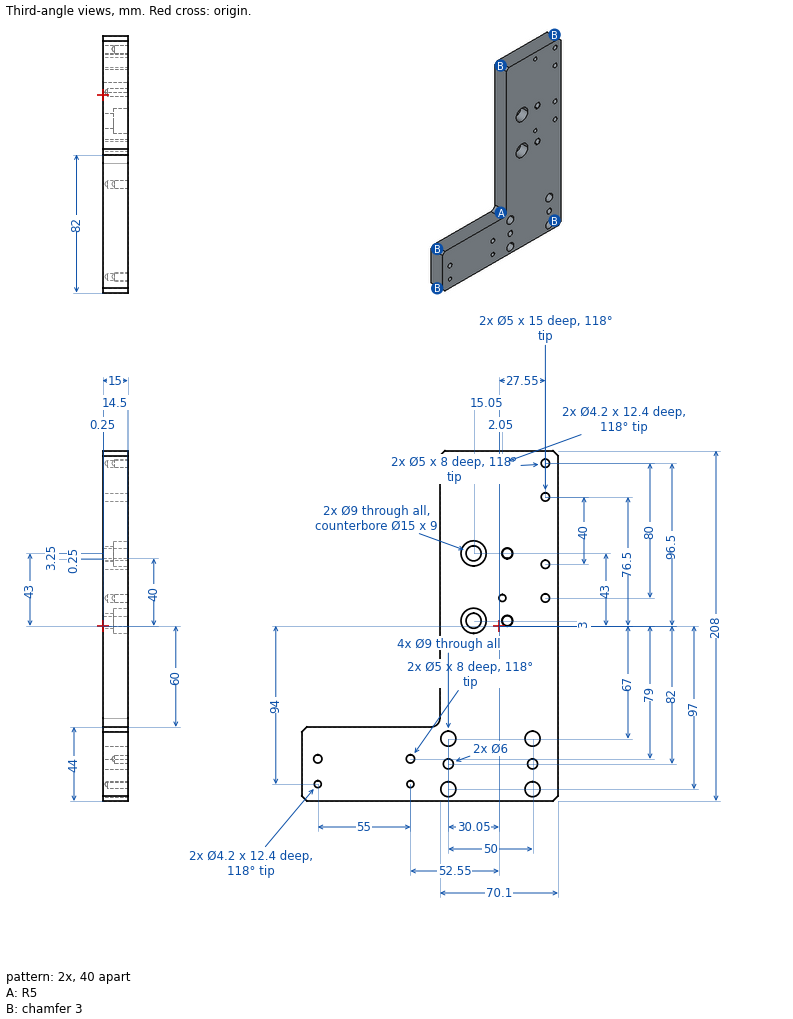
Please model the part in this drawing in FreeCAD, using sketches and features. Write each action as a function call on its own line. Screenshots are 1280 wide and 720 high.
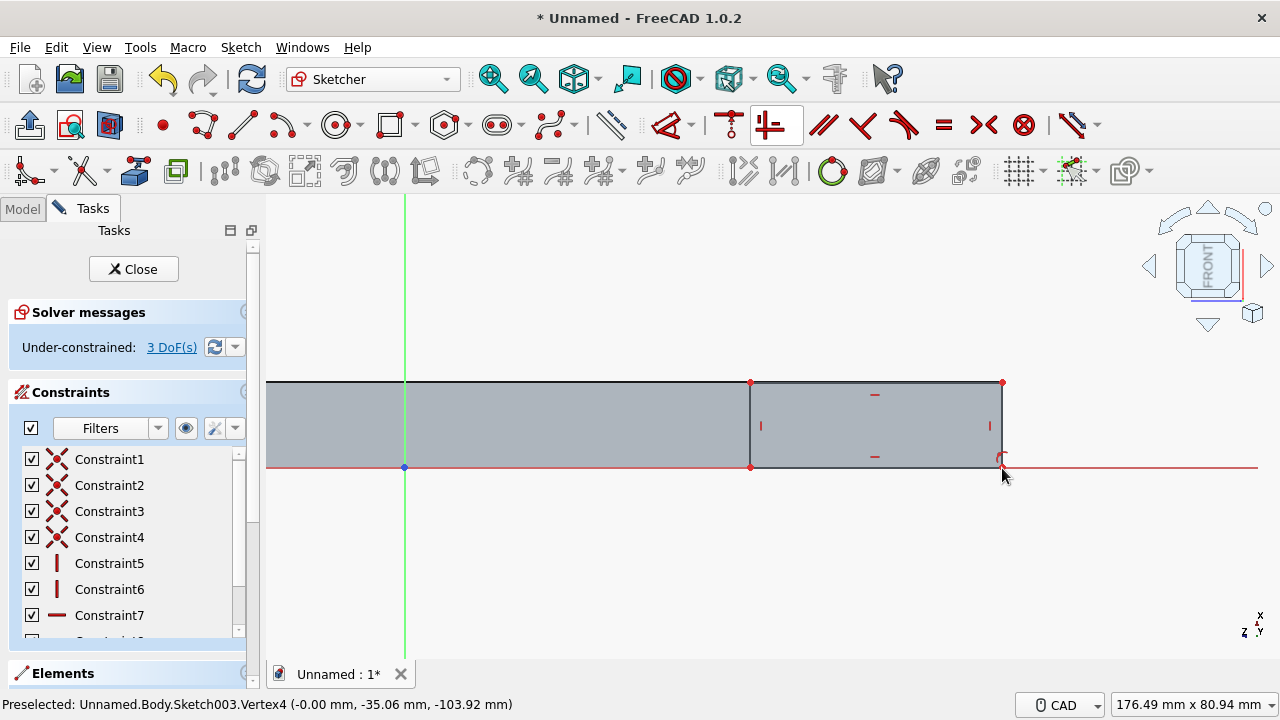
key(d)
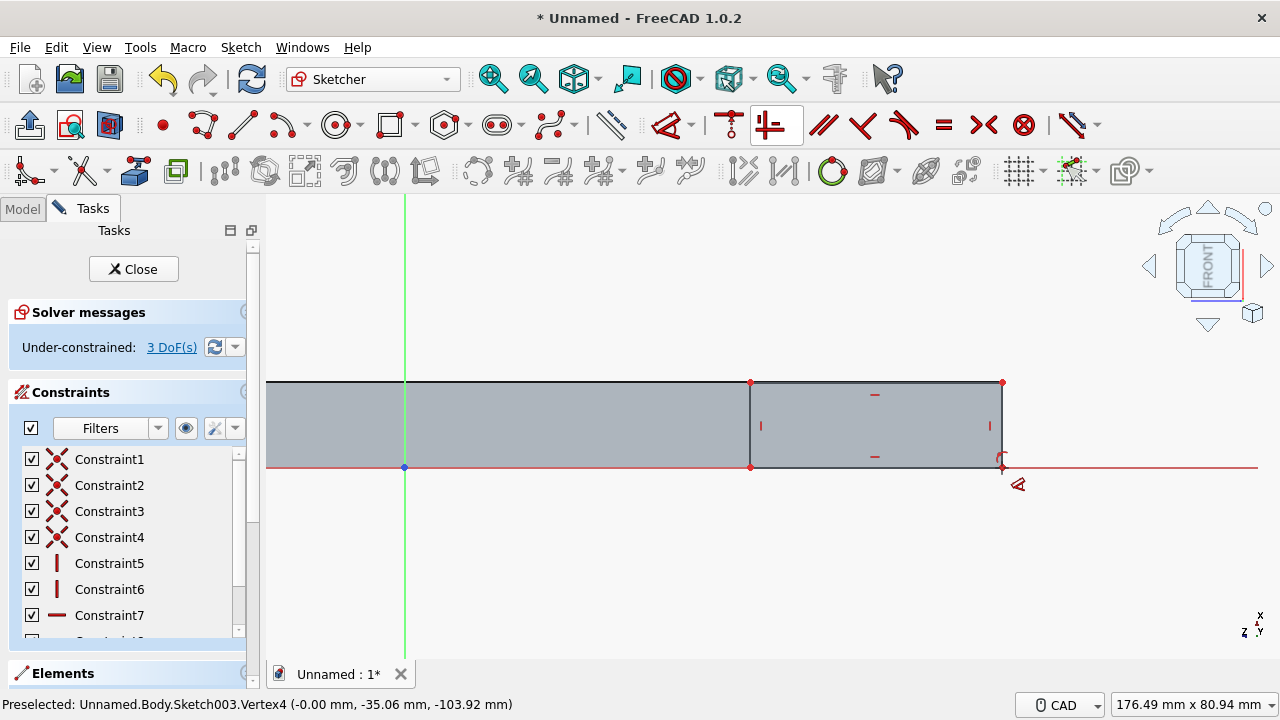
click(750, 408)
click(784, 425)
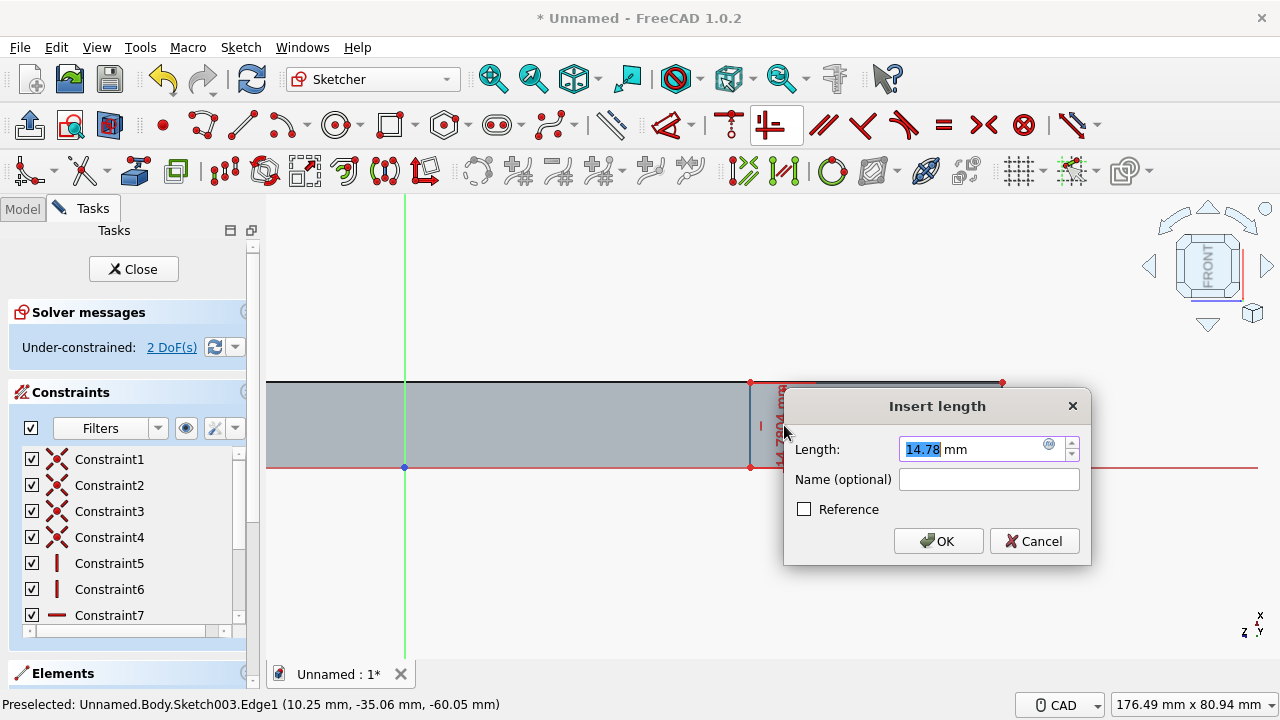
text(15)
key(Return)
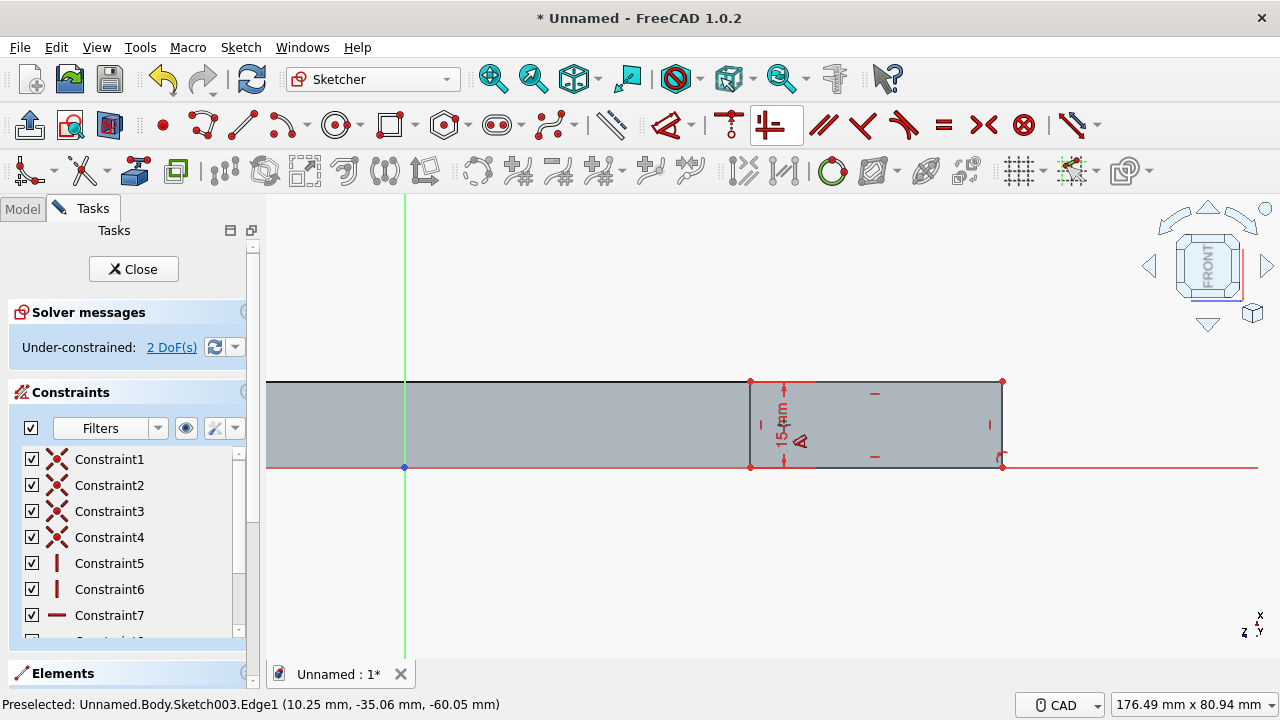
click(826, 468)
click(876, 502)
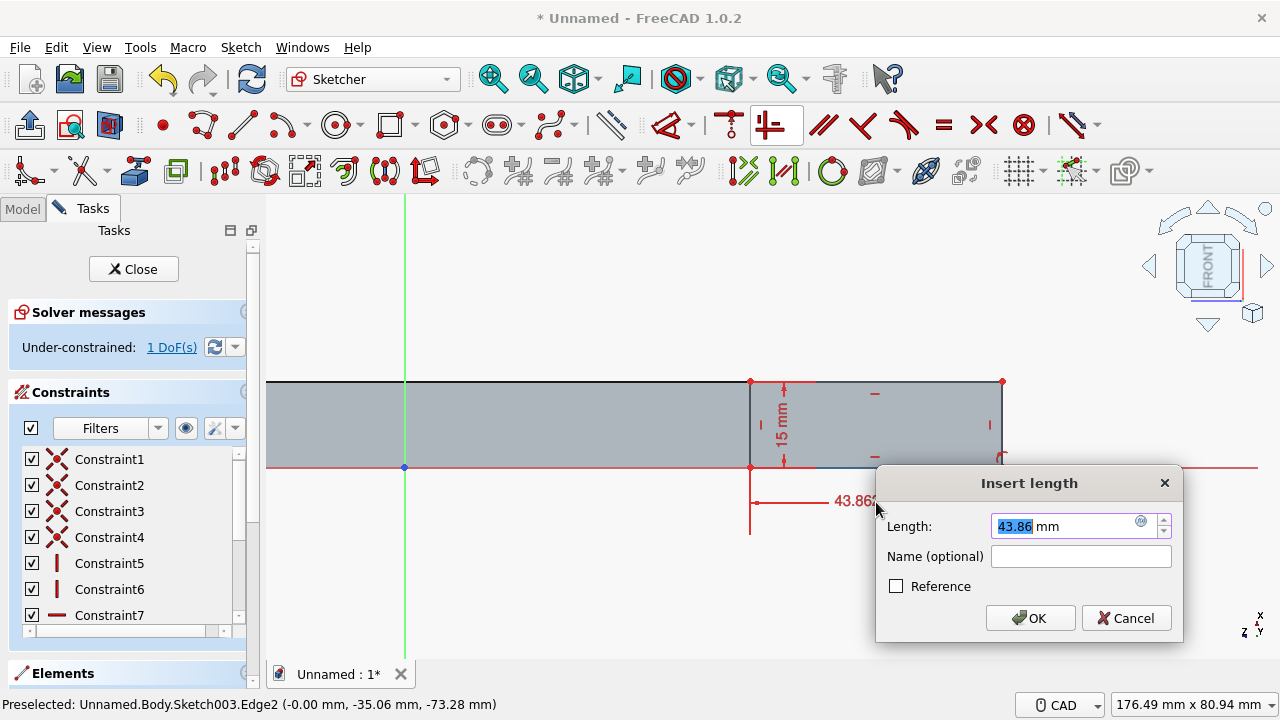
text(44)
key(Return)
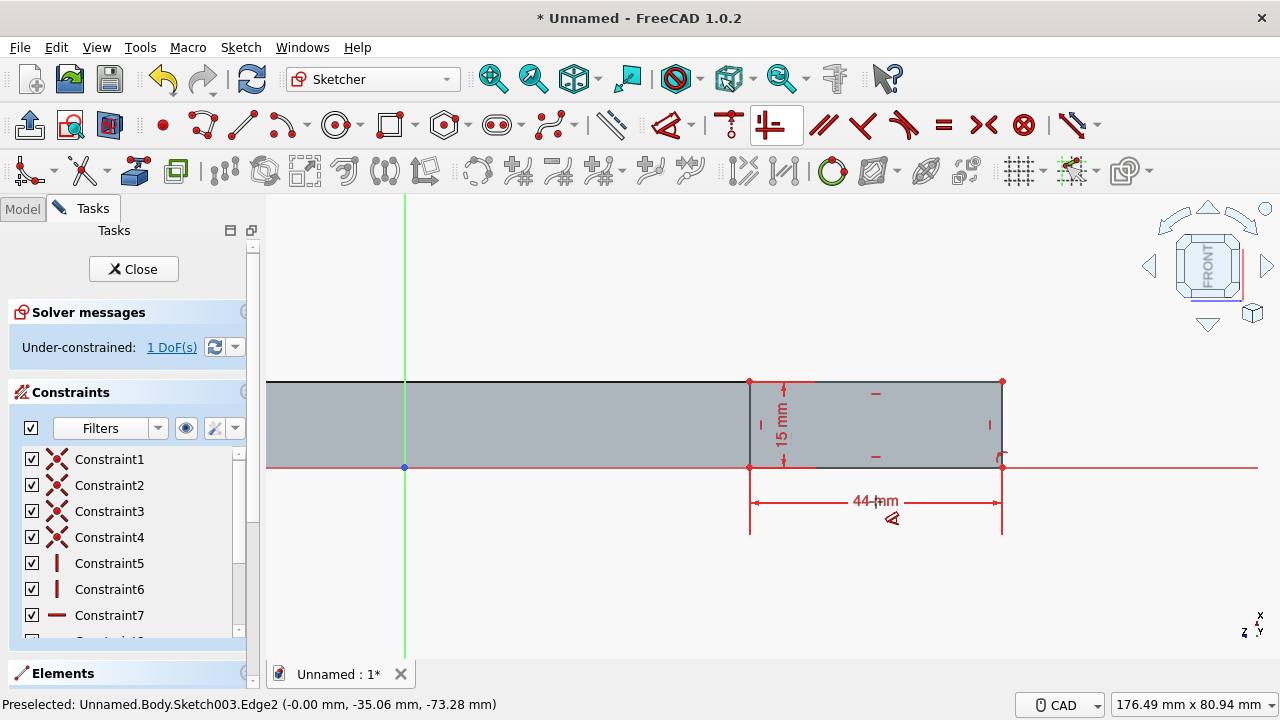
click(750, 382)
click(577, 502)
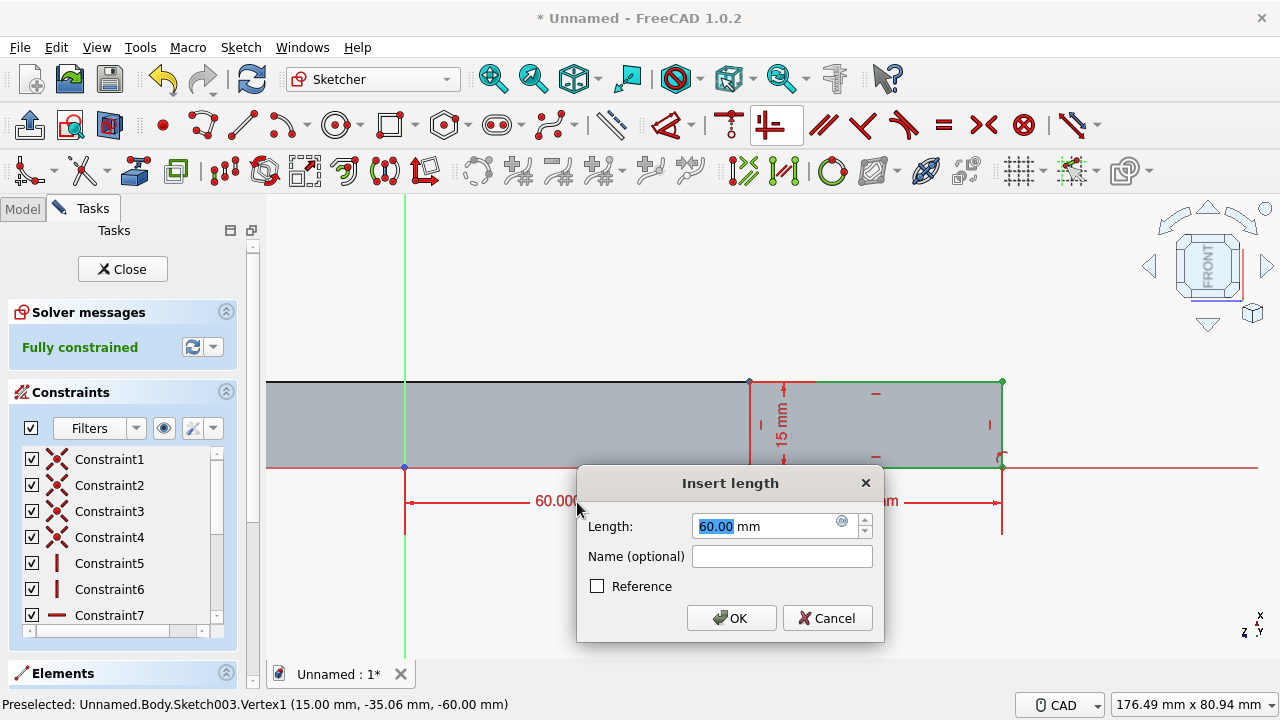
text(60)
key(Return)
key(Escape)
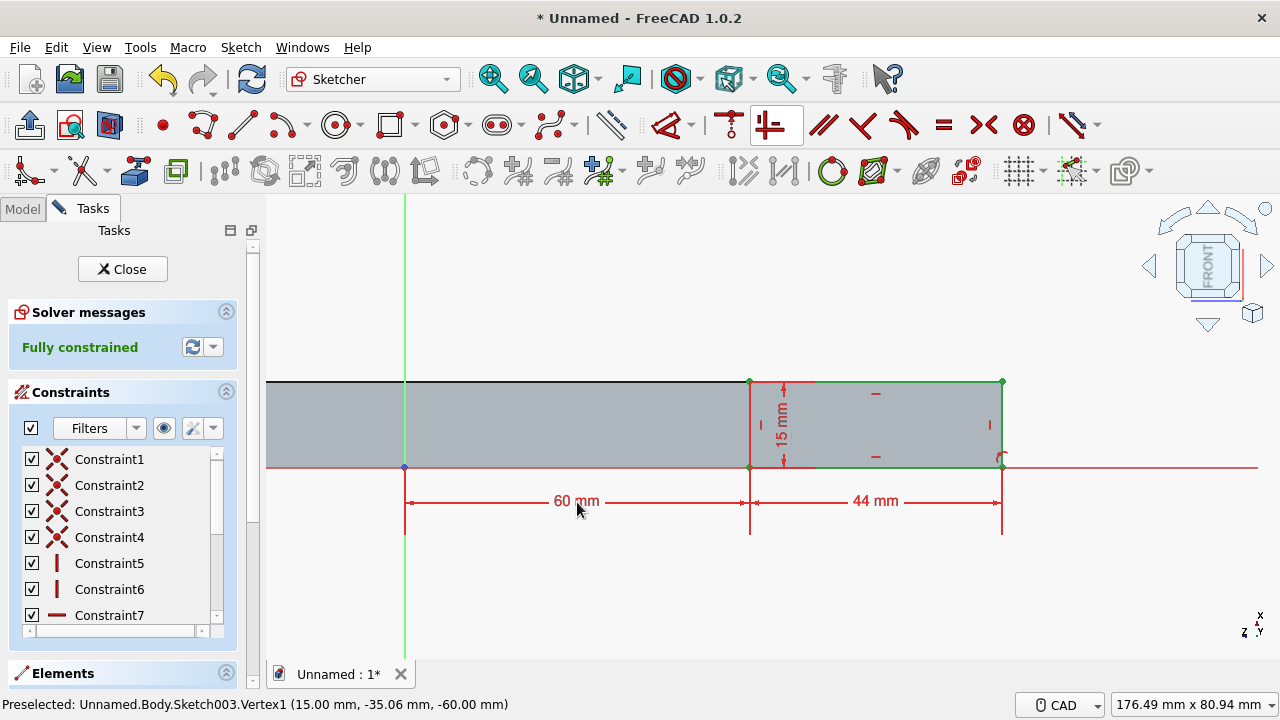
click(123, 269)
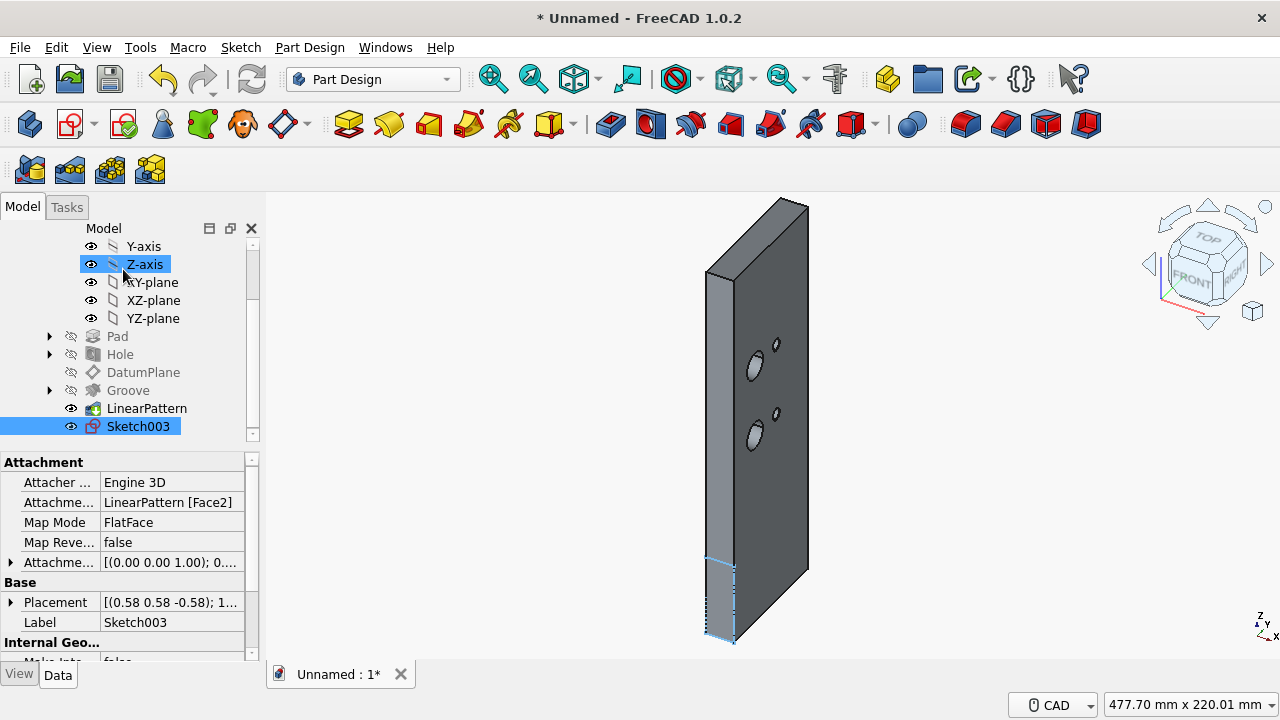
click(350, 124)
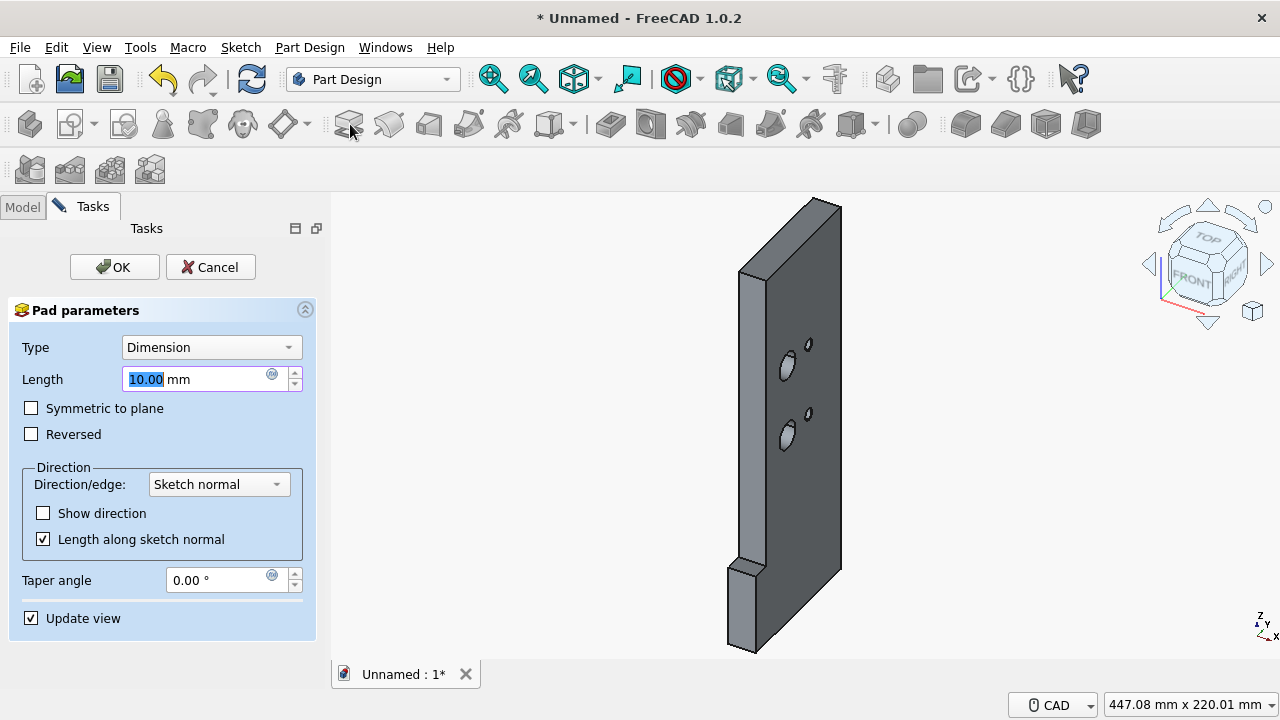
text(82)
key(Tab)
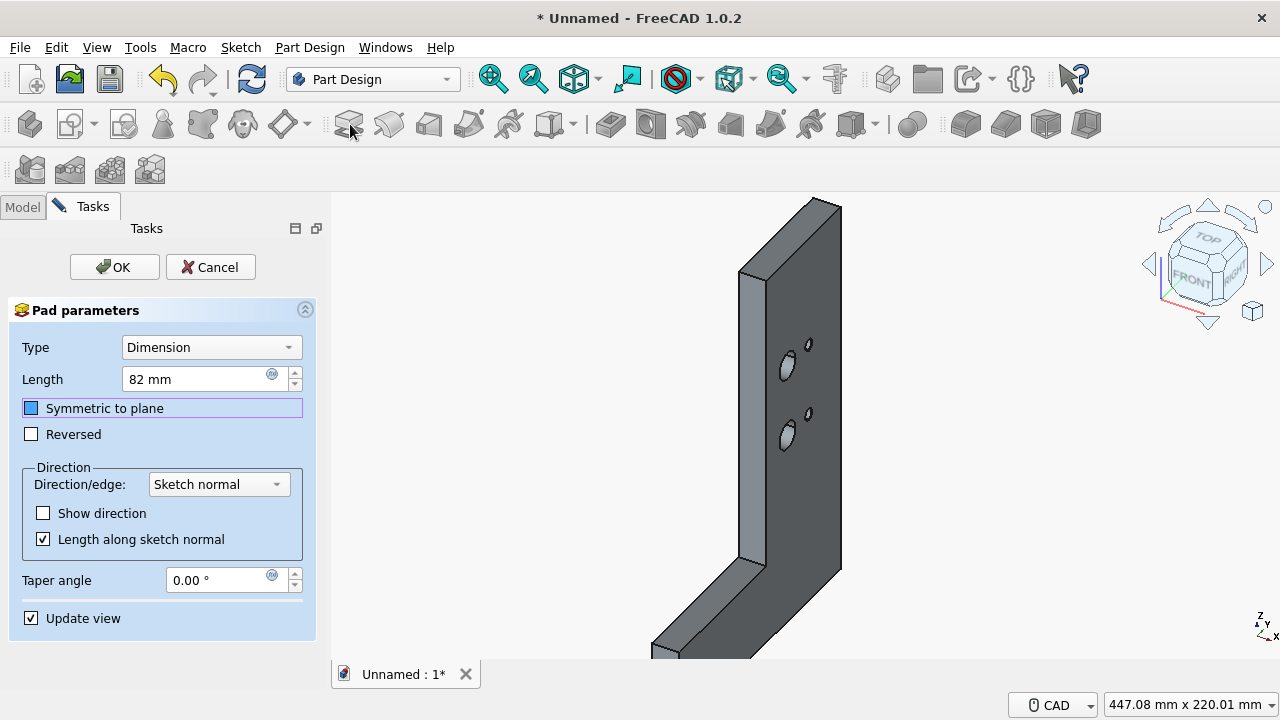
click(115, 267)